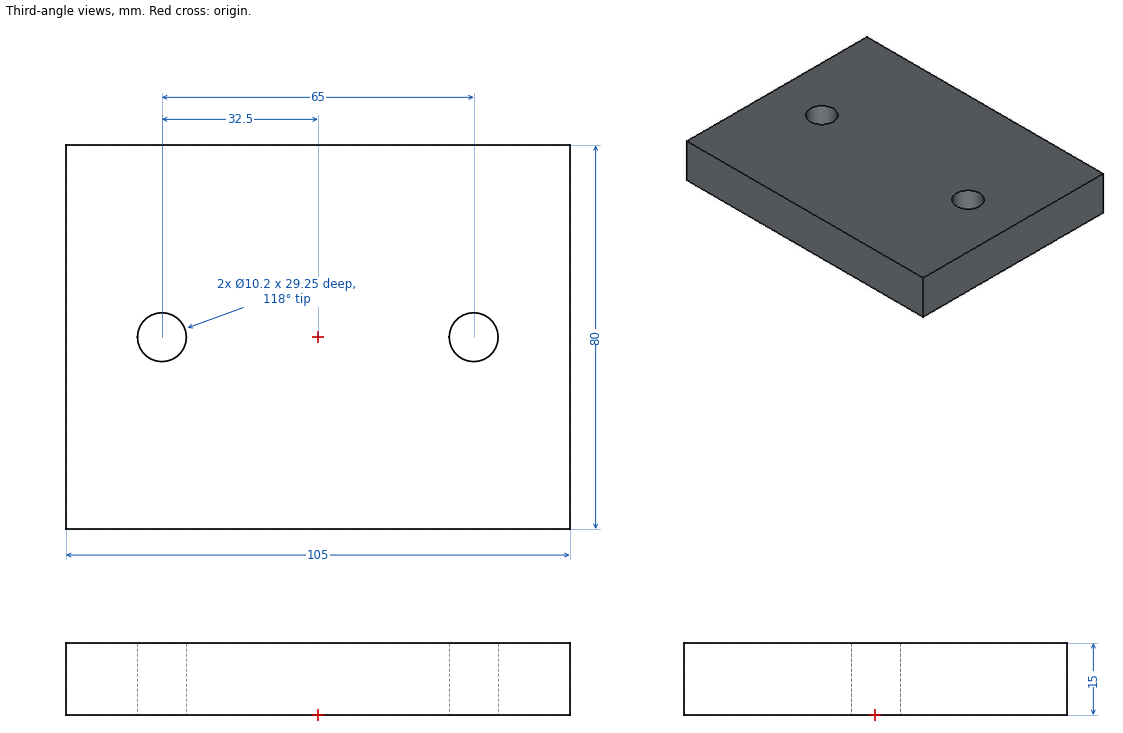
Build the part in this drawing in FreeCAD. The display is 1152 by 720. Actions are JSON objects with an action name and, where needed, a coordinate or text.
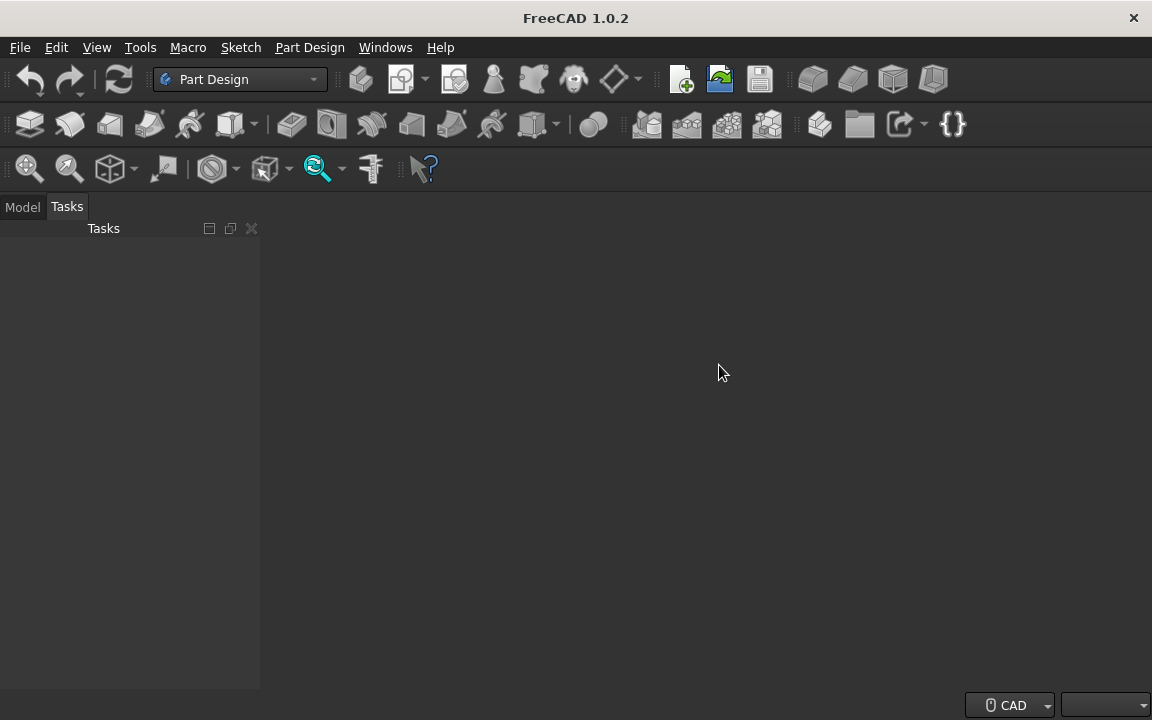
{"action": "left_click", "coordinate": [680, 80]}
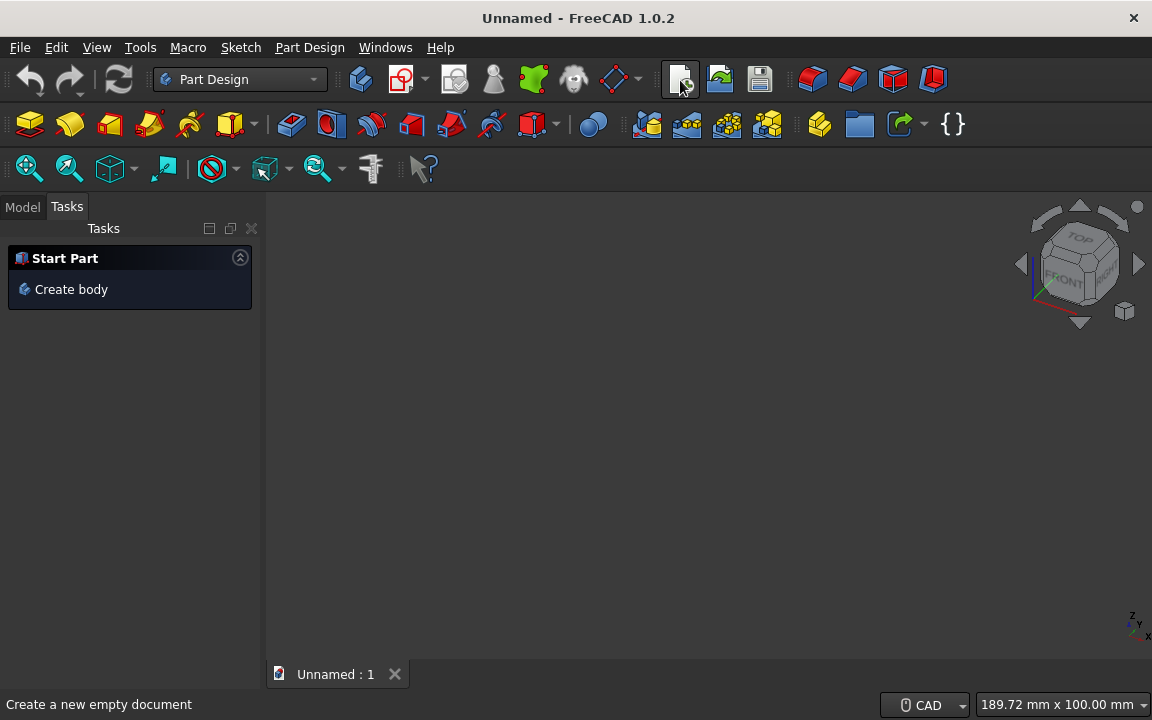
{"action": "left_click", "coordinate": [402, 80]}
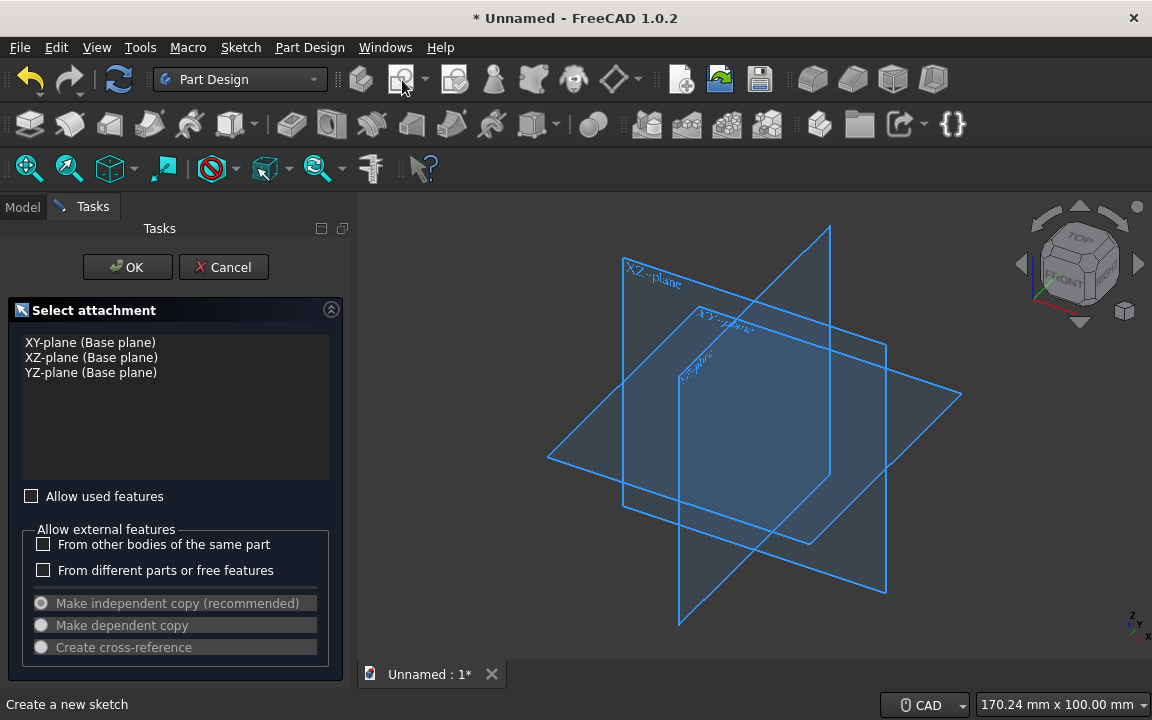
{"action": "left_click", "coordinate": [82, 342]}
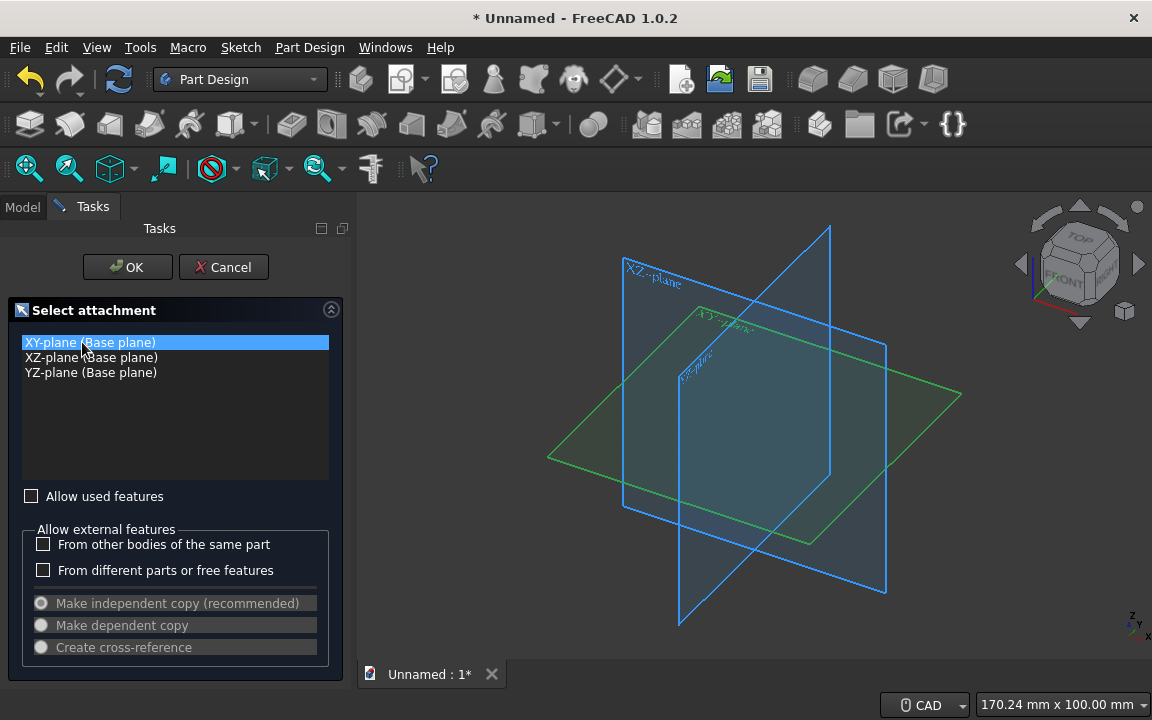
{"action": "left_click", "coordinate": [128, 267]}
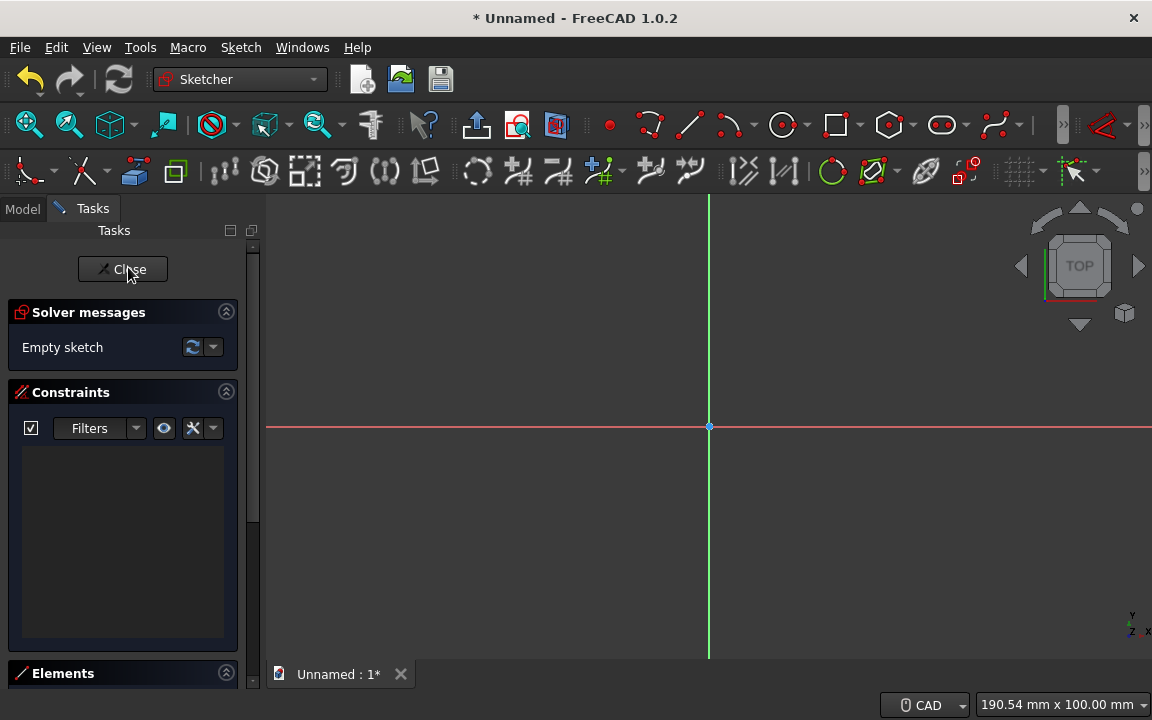
{"action": "scroll", "coordinate": [331, 427], "scroll_direction": "down", "scroll_amount": 1}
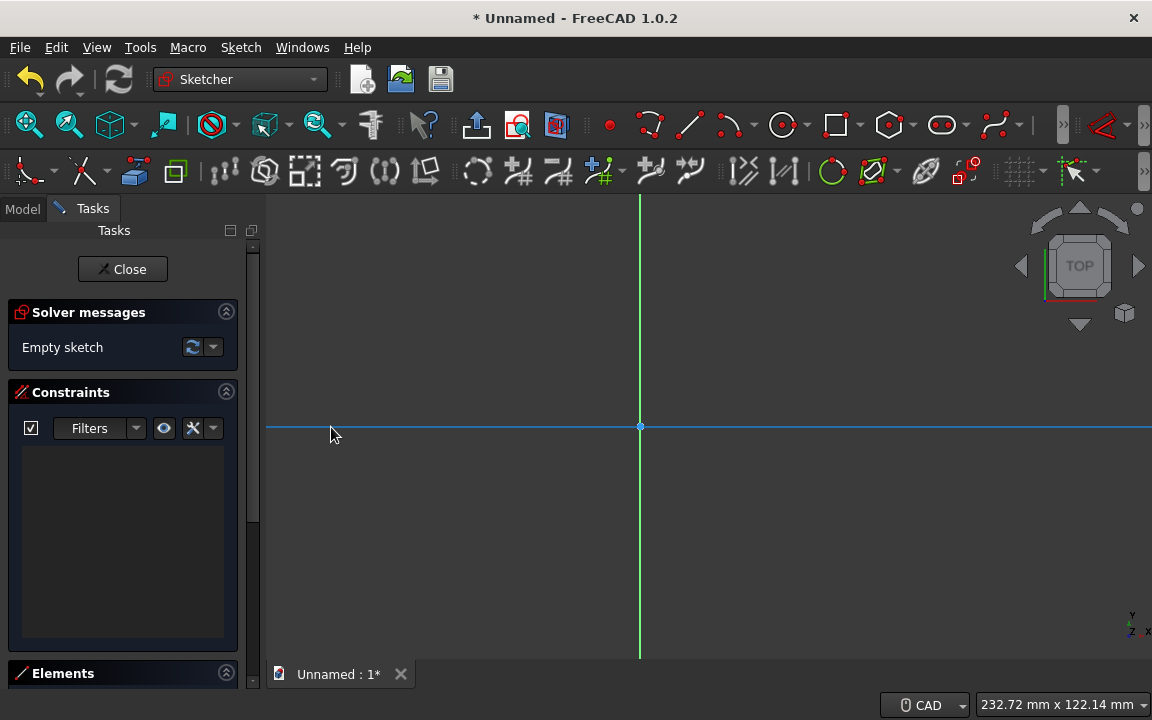
{"action": "left_click", "coordinate": [862, 126]}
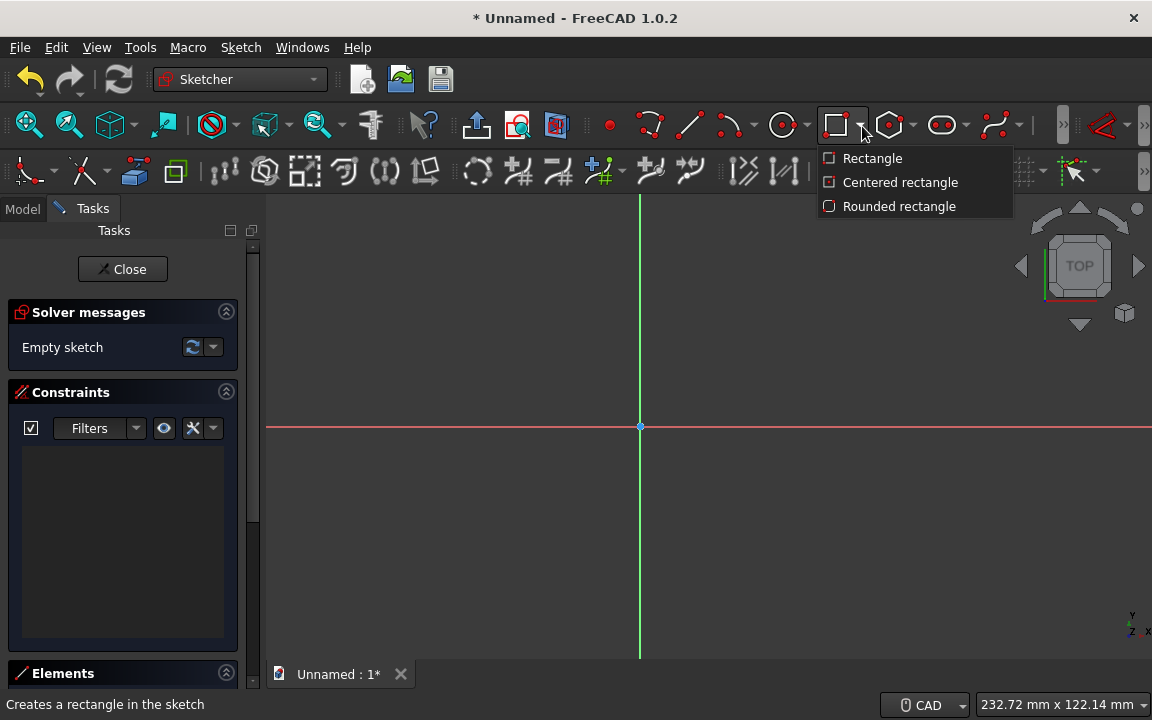
{"action": "left_click", "coordinate": [916, 182]}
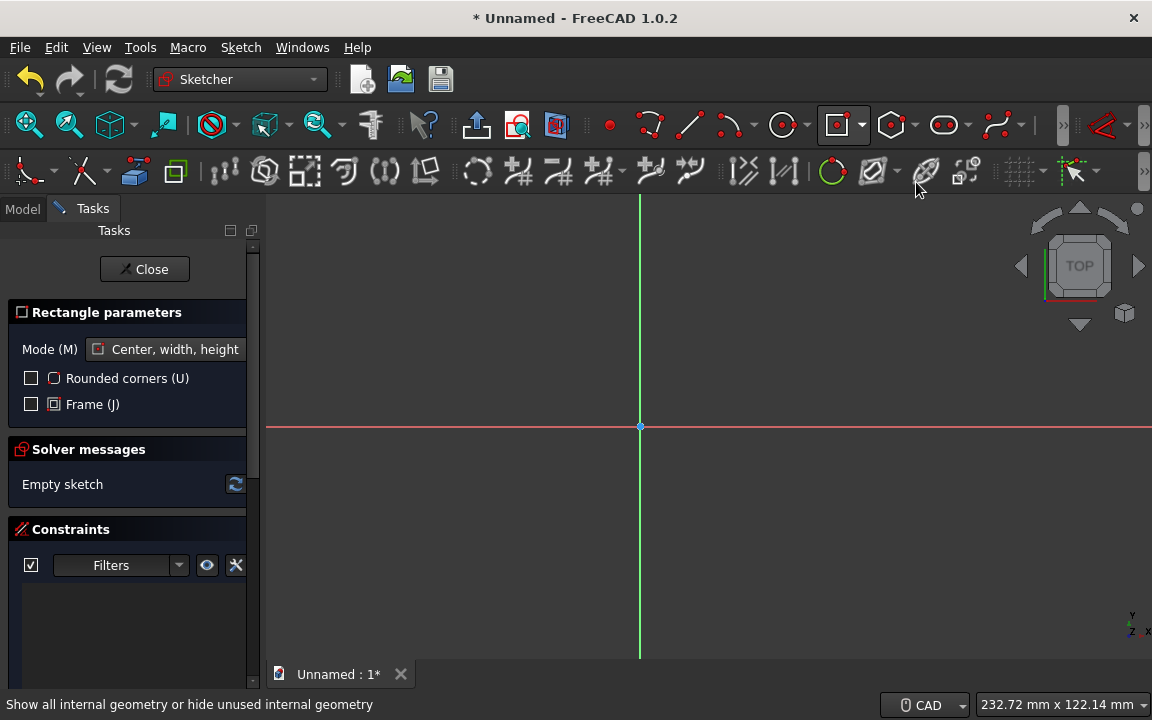
{"action": "left_click", "coordinate": [640, 427]}
{"action": "mouse_move", "coordinate": [840, 274]}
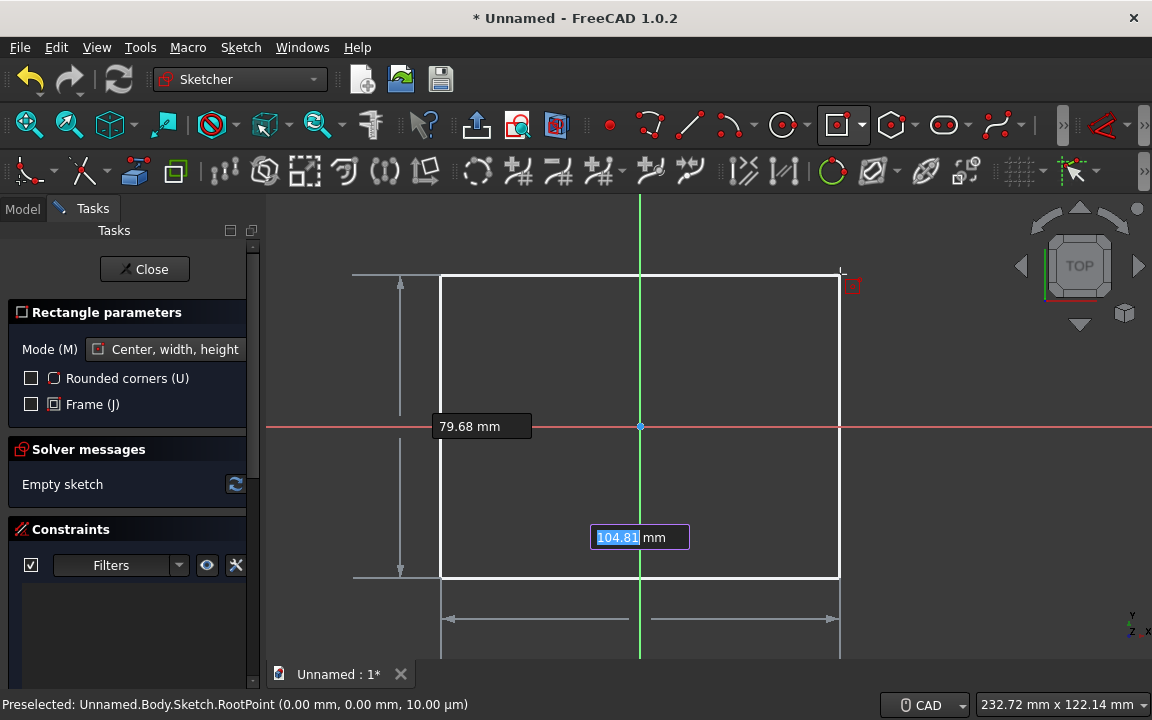
{"action": "type", "text": "105"}
{"action": "key", "text": "Tab"}
{"action": "type", "text": "80"}
{"action": "key", "text": "Return"}
{"action": "key", "text": "Escape"}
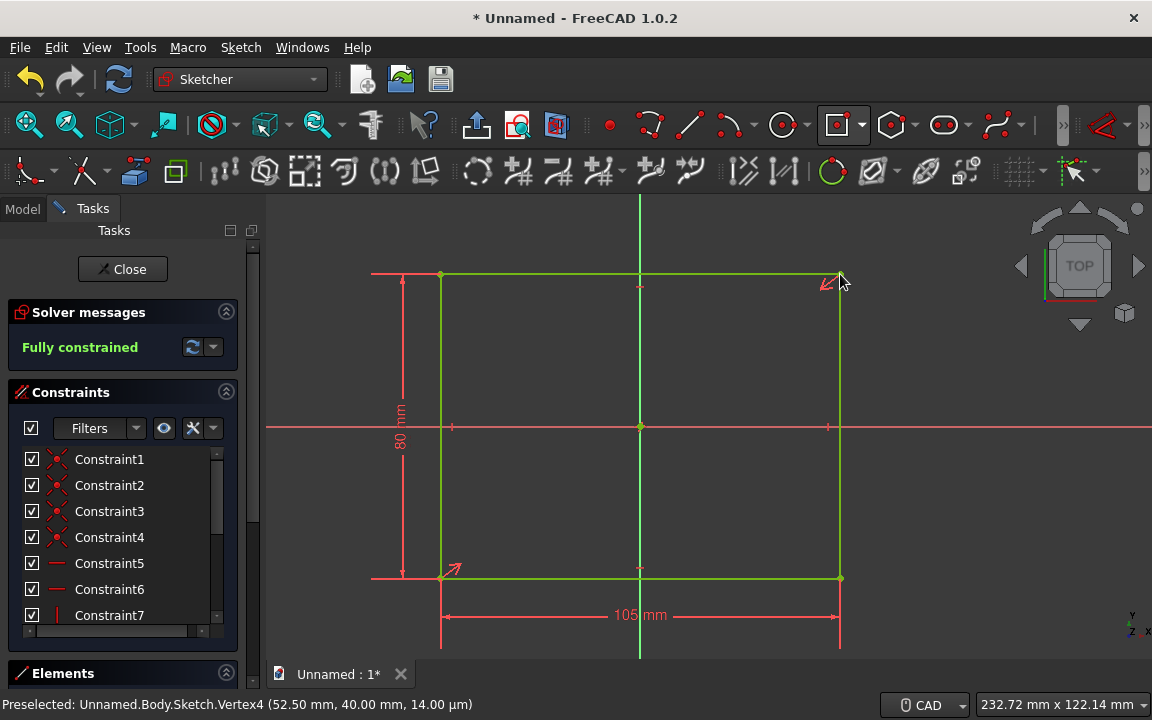
{"action": "left_click", "coordinate": [123, 269]}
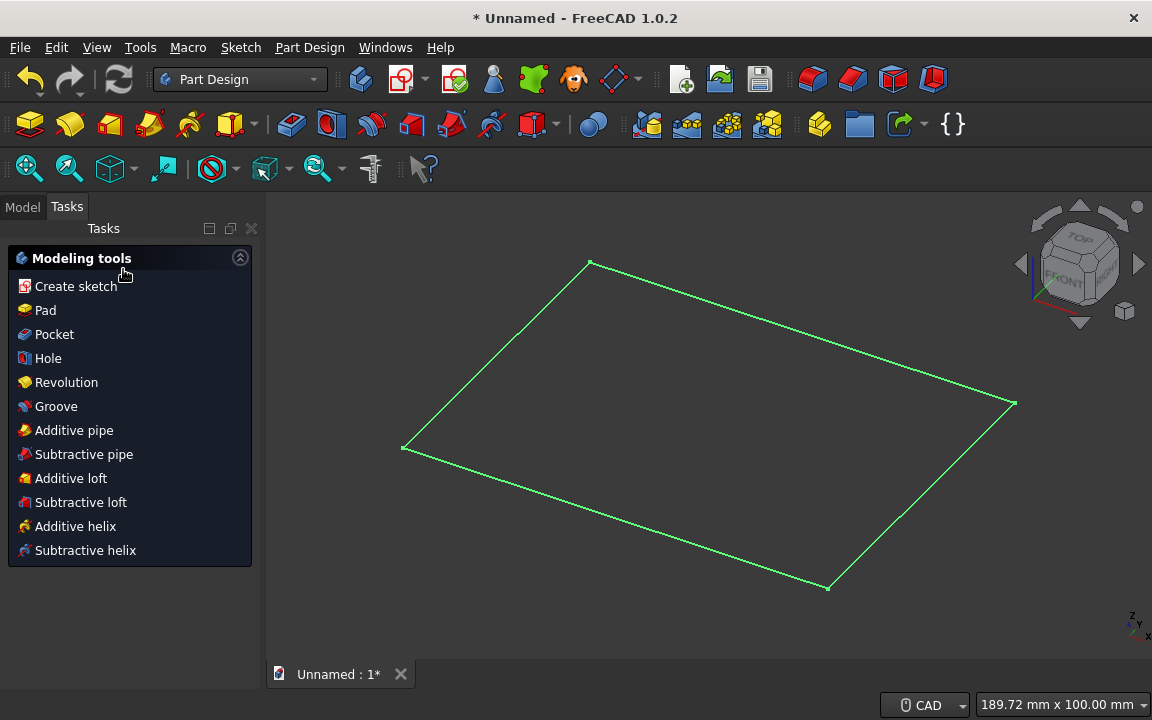
{"action": "left_click", "coordinate": [30, 124]}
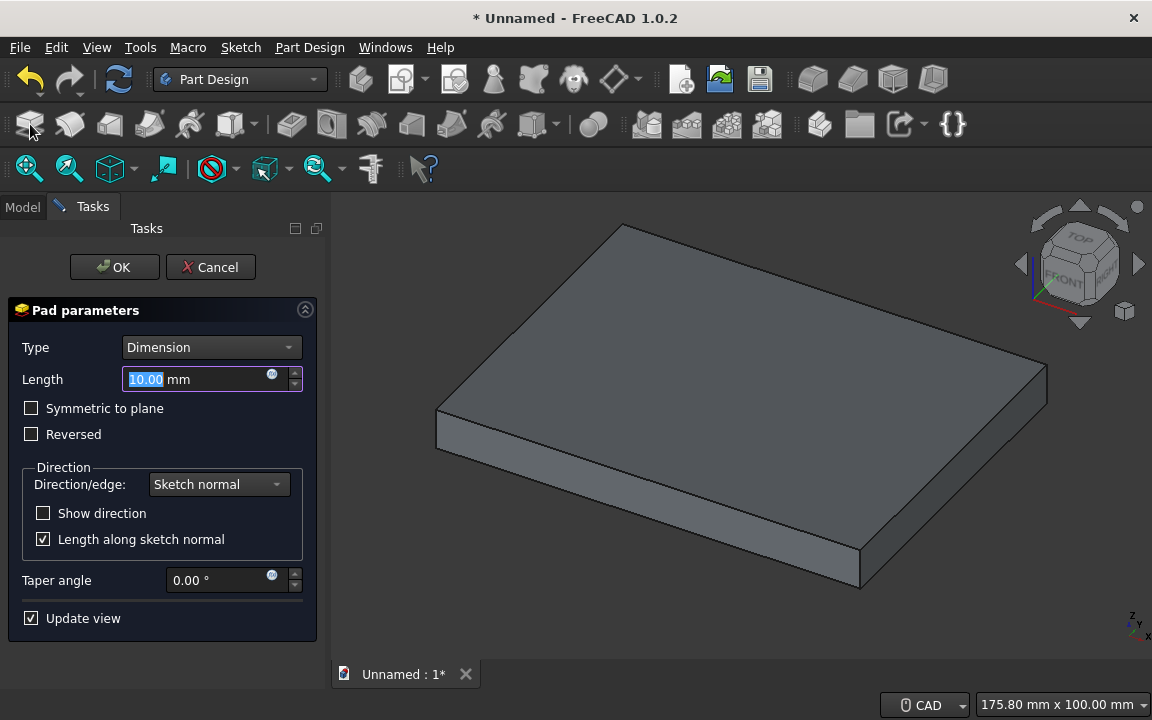
{"action": "type", "text": "15"}
{"action": "key", "text": "Tab"}